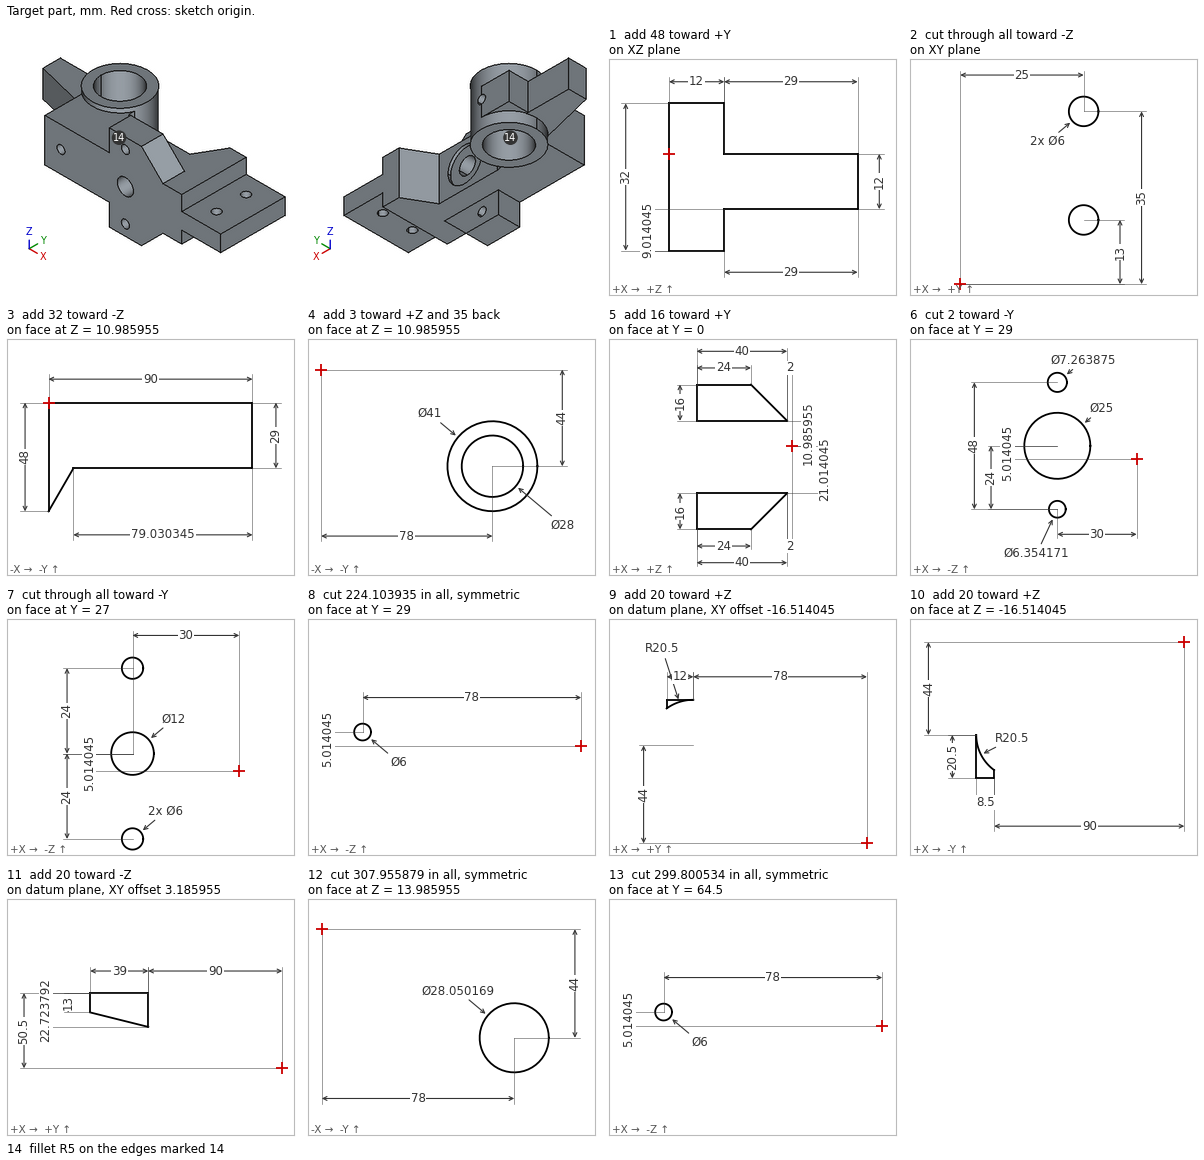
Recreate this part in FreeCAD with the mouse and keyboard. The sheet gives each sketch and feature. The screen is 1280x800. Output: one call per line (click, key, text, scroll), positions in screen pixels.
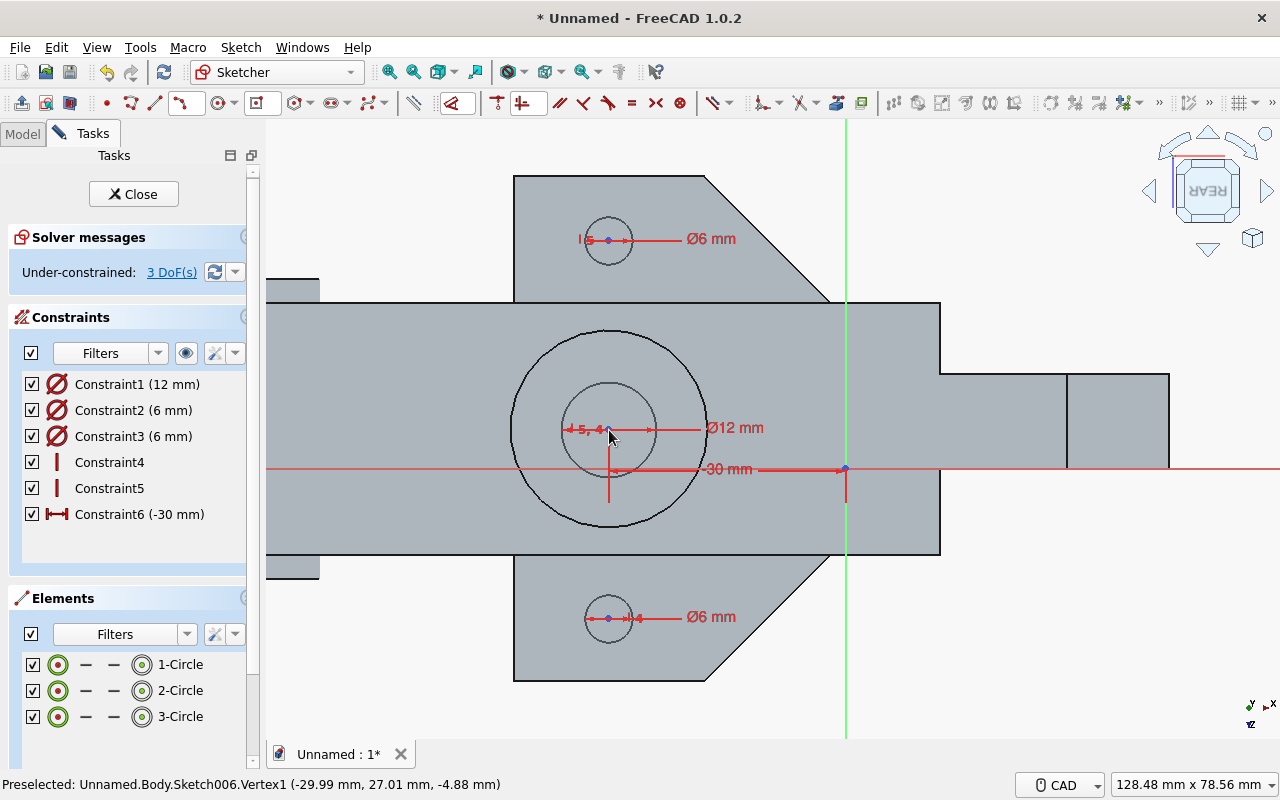
click(609, 430)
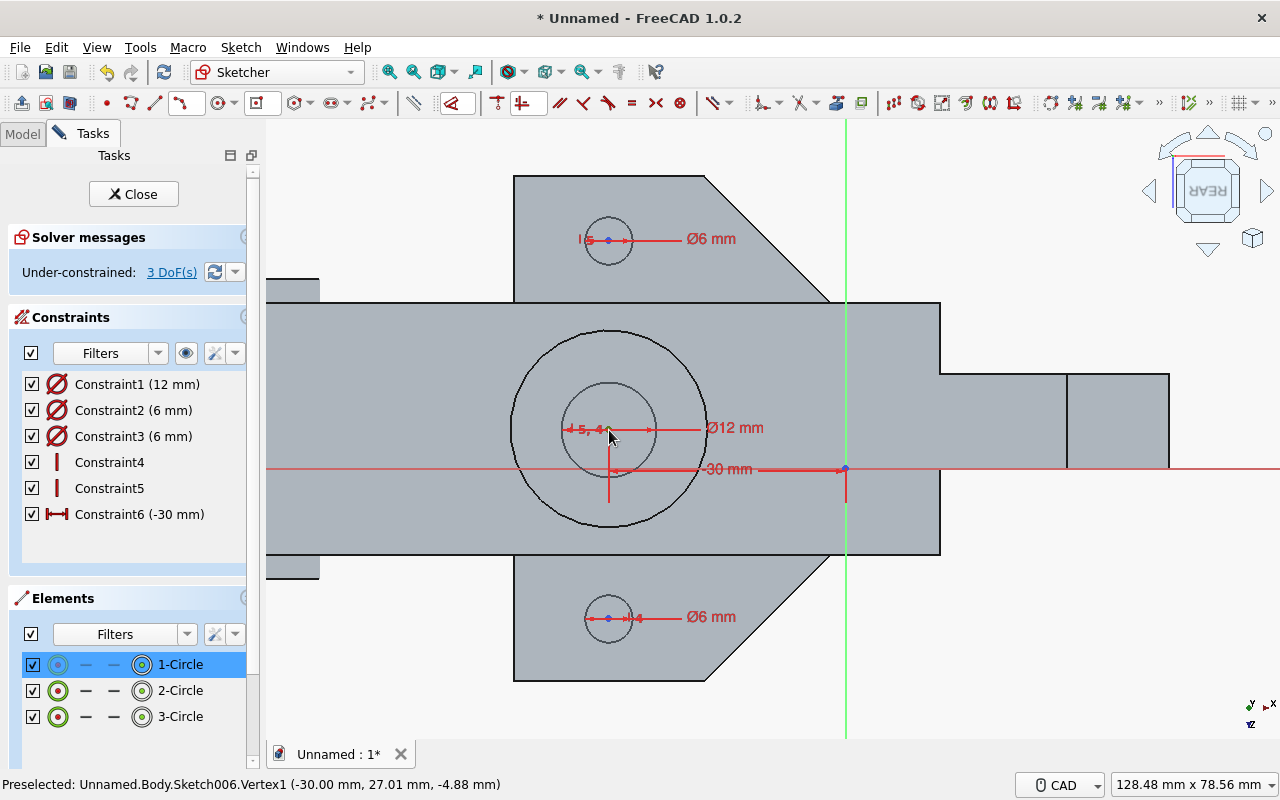
click(609, 619)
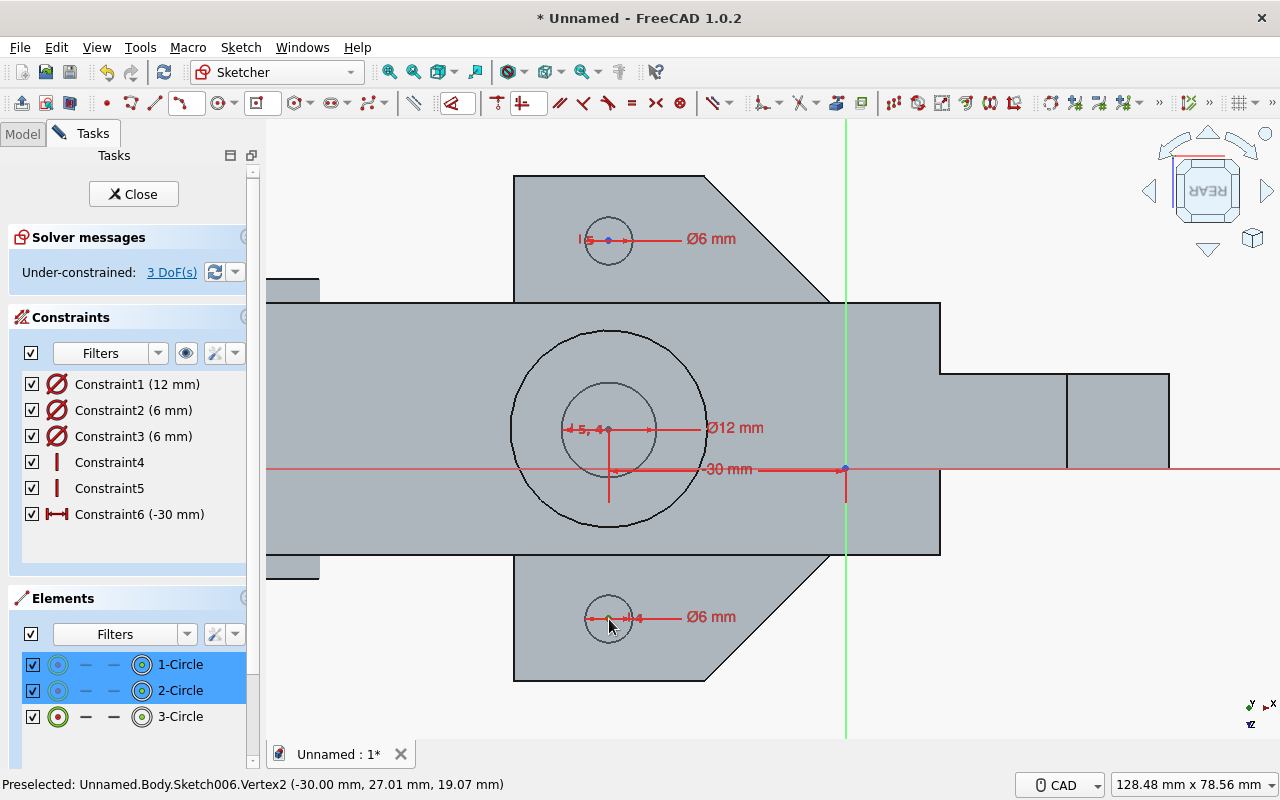
key(i)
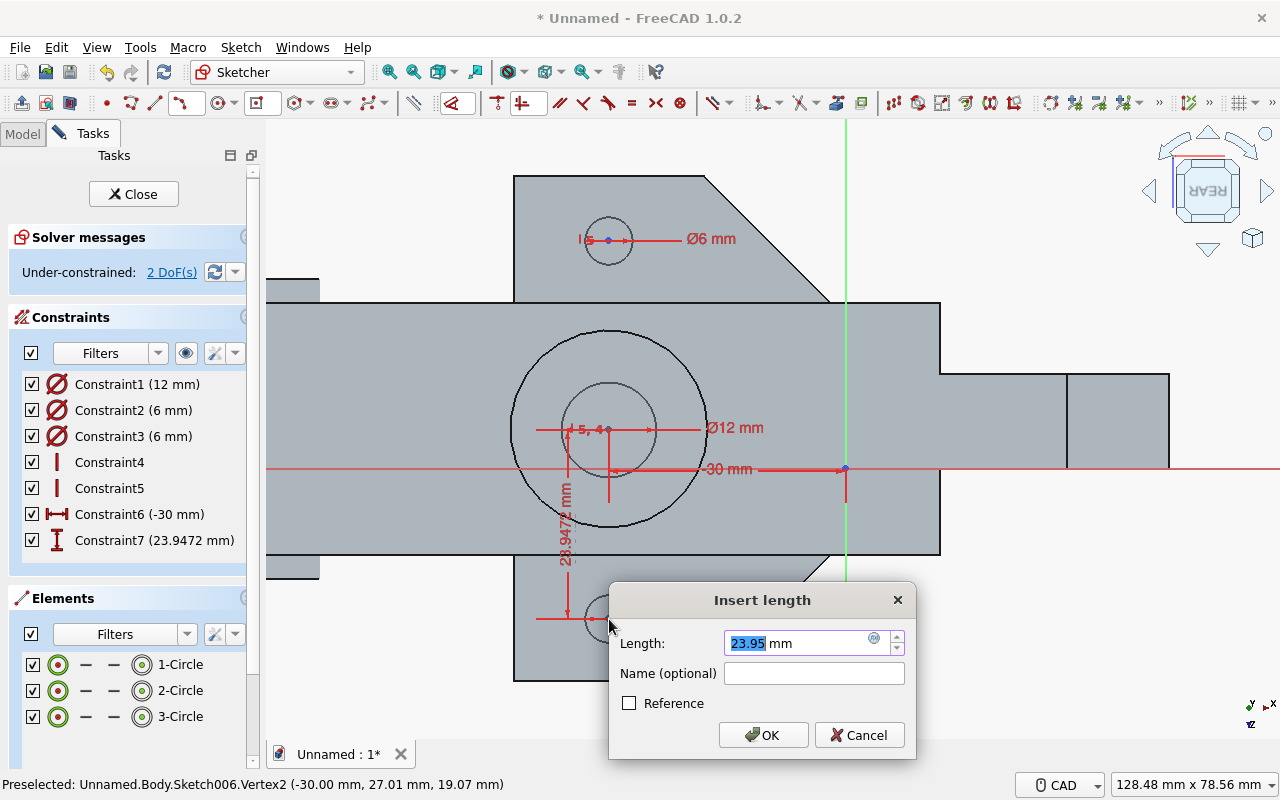
text(24)
key(Return)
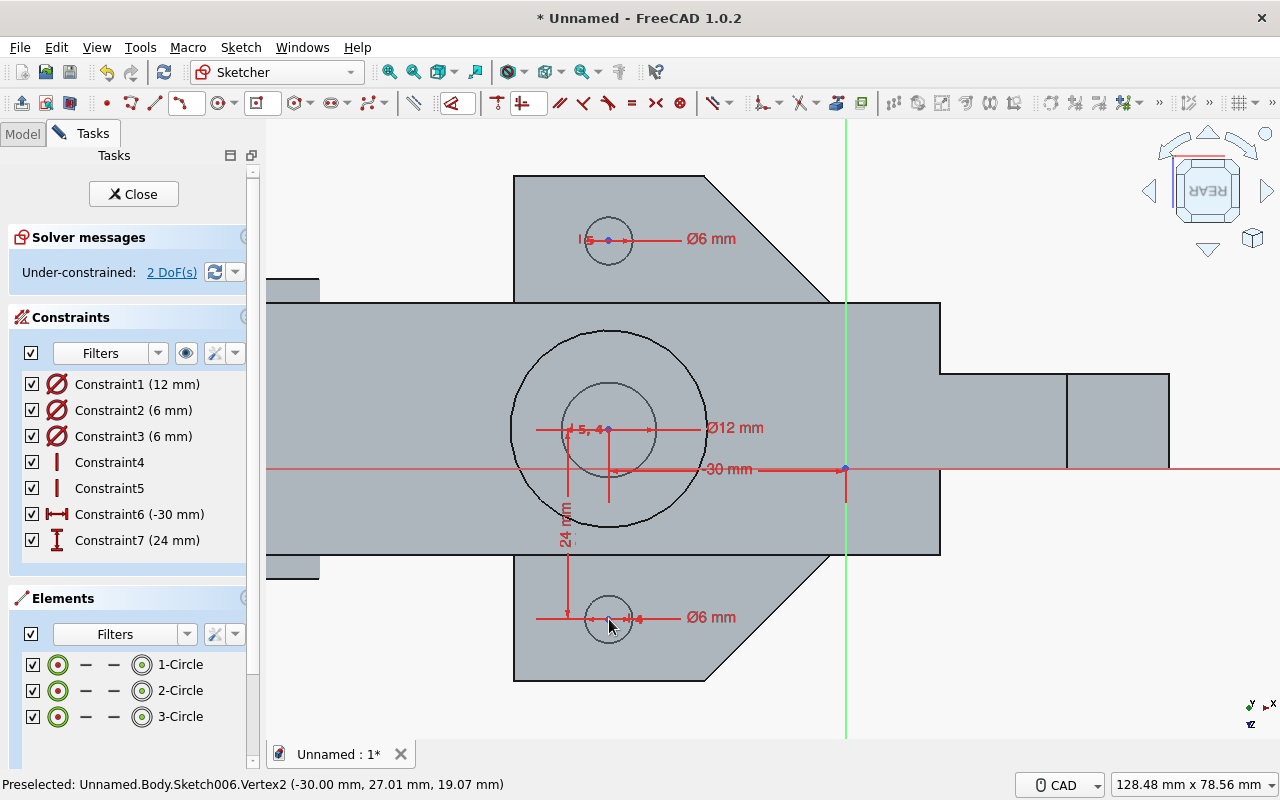
click(609, 430)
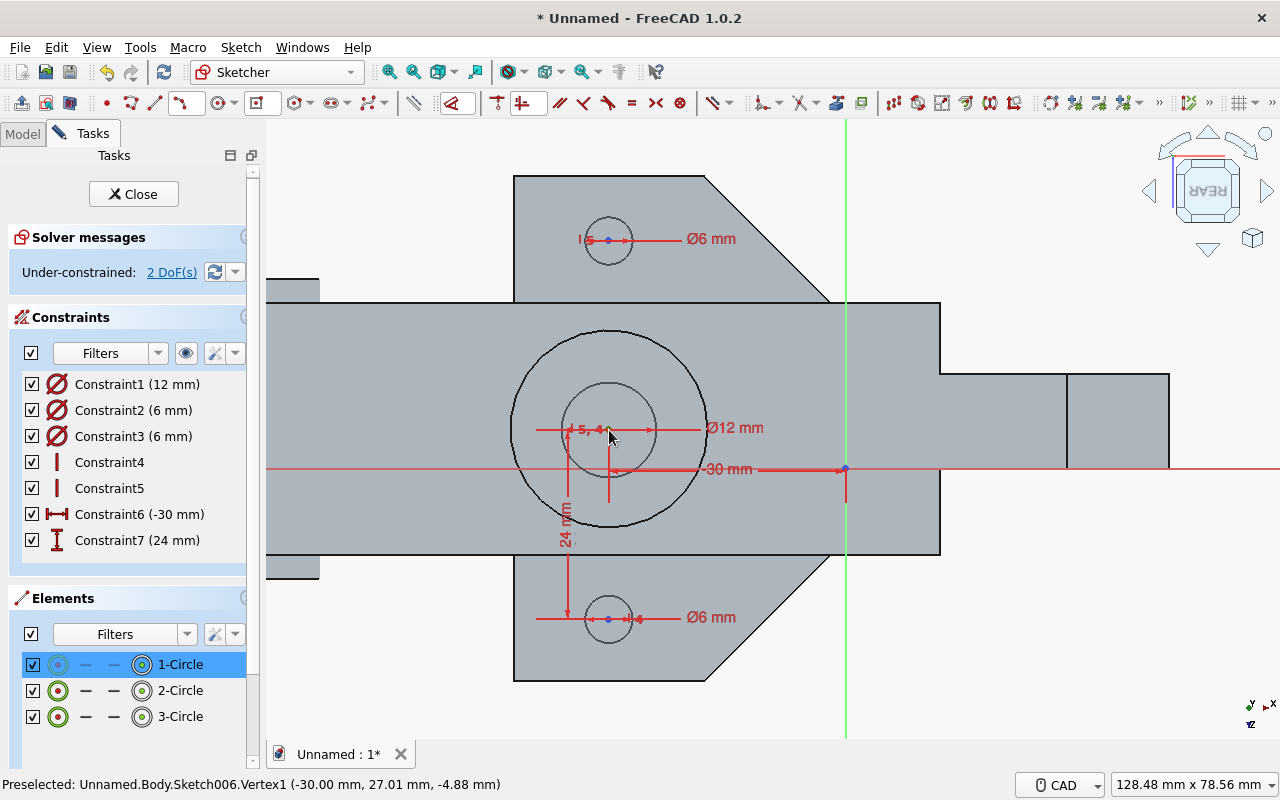
click(609, 241)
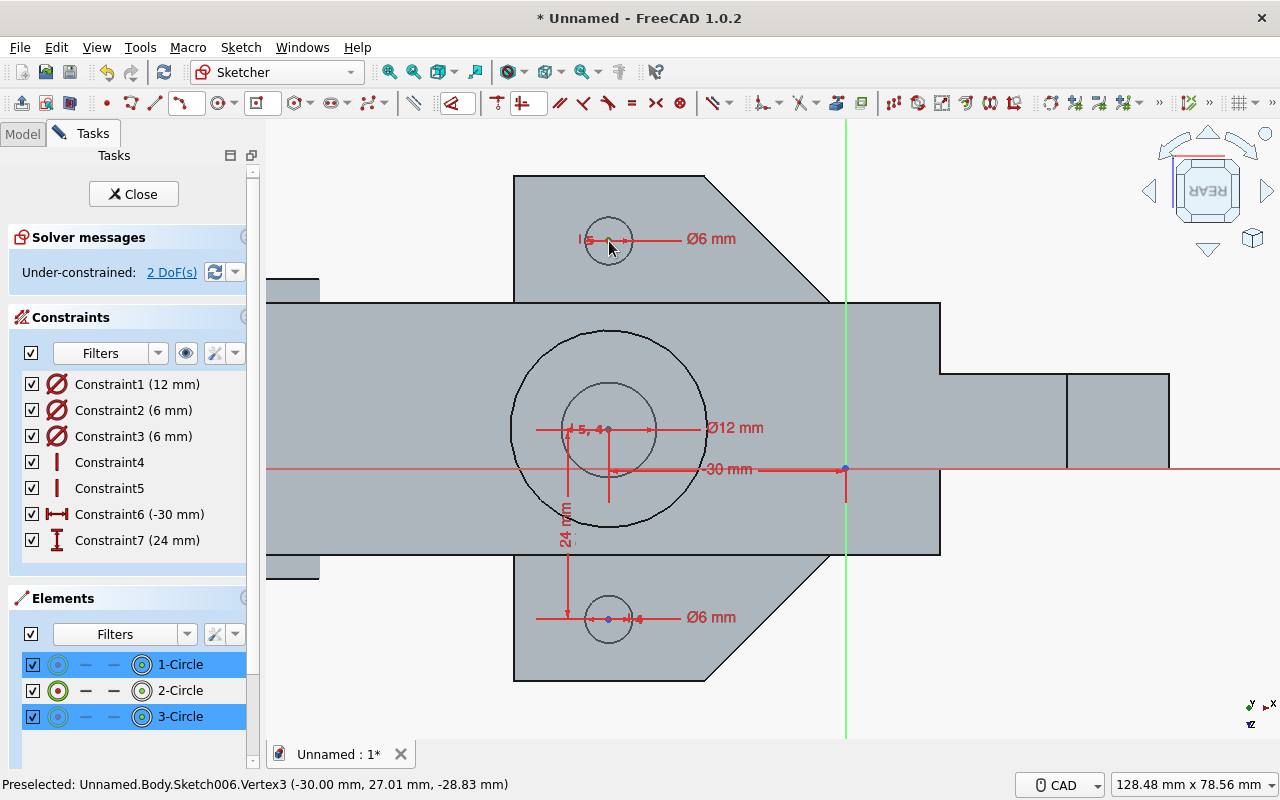
key(i)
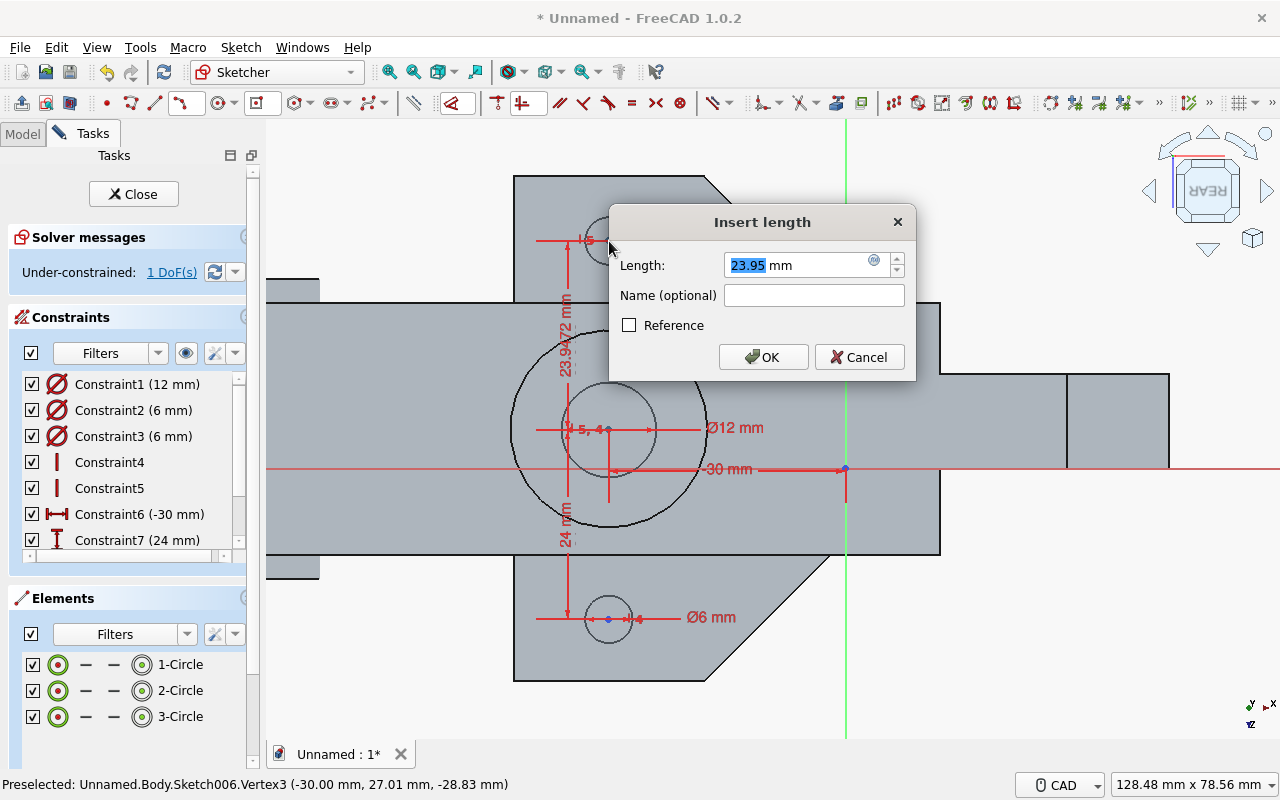
text(24)
key(Return)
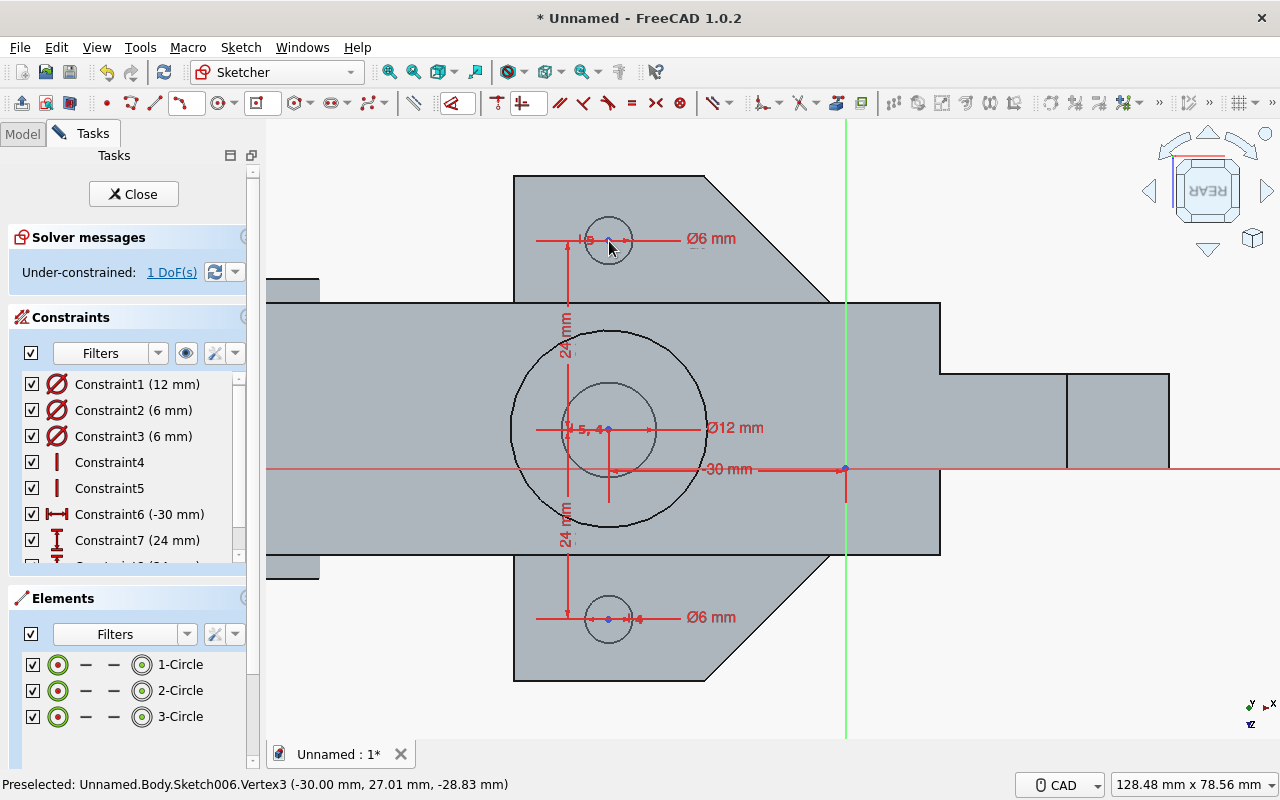
click(609, 430)